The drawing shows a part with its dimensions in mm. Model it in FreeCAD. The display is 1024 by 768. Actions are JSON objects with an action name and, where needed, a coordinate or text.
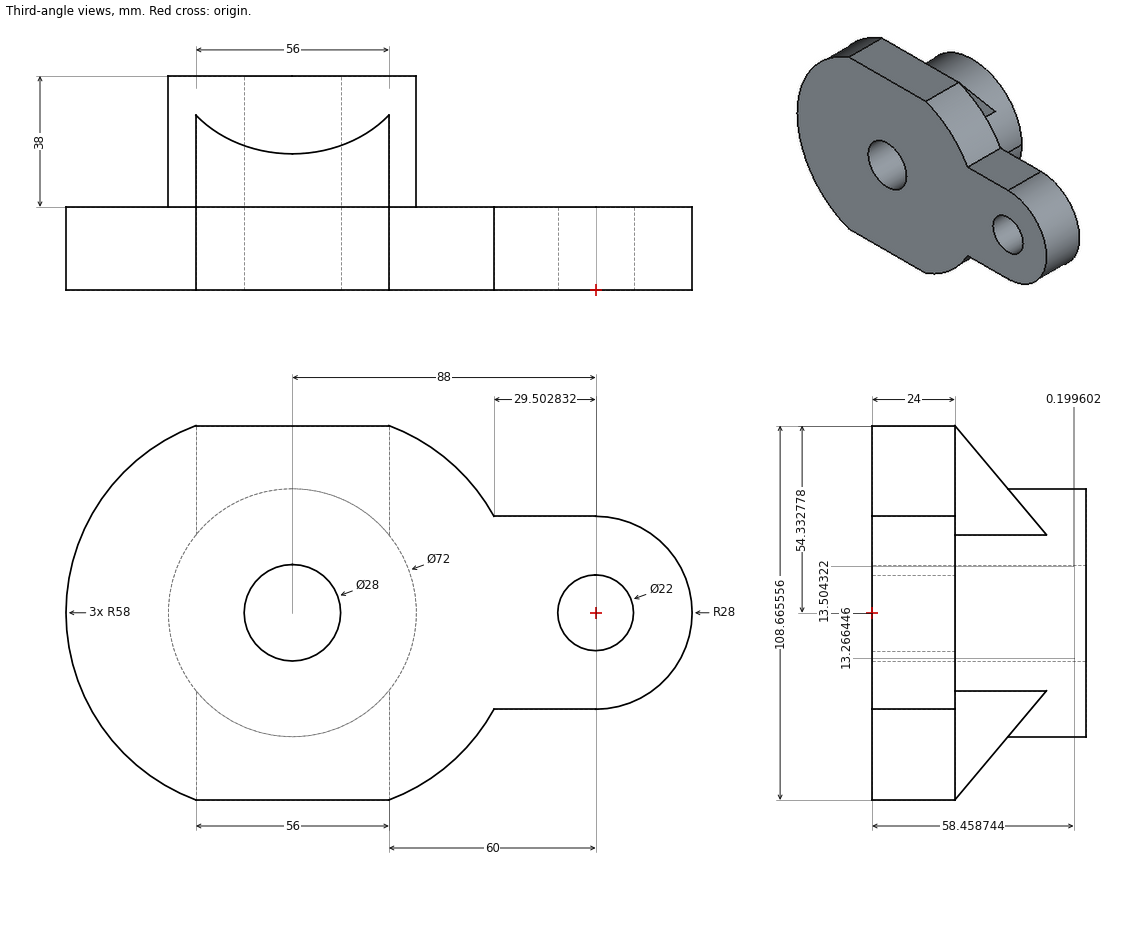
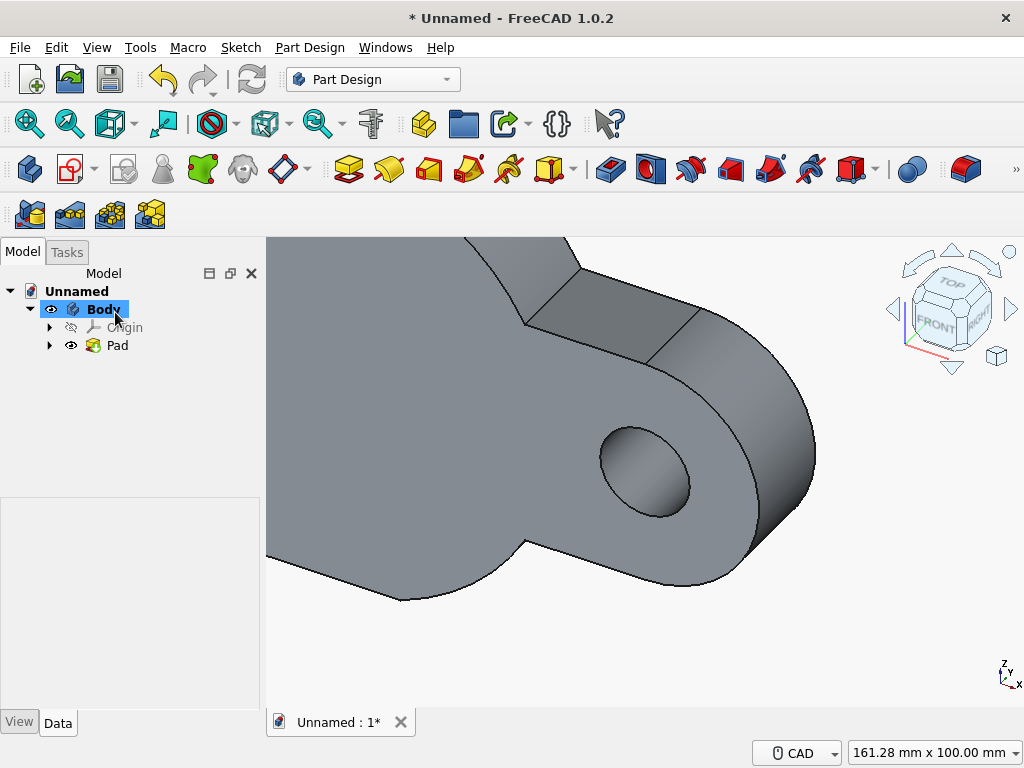
{"action": "left_click", "coordinate": [30, 124]}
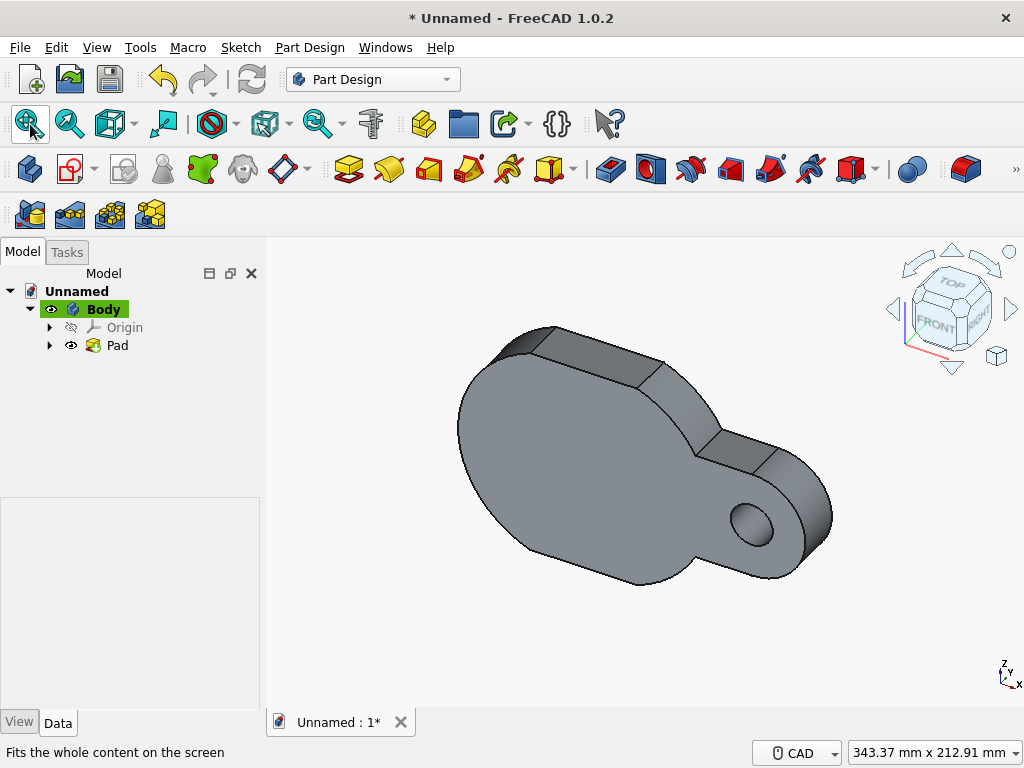
{"action": "key", "text": "4"}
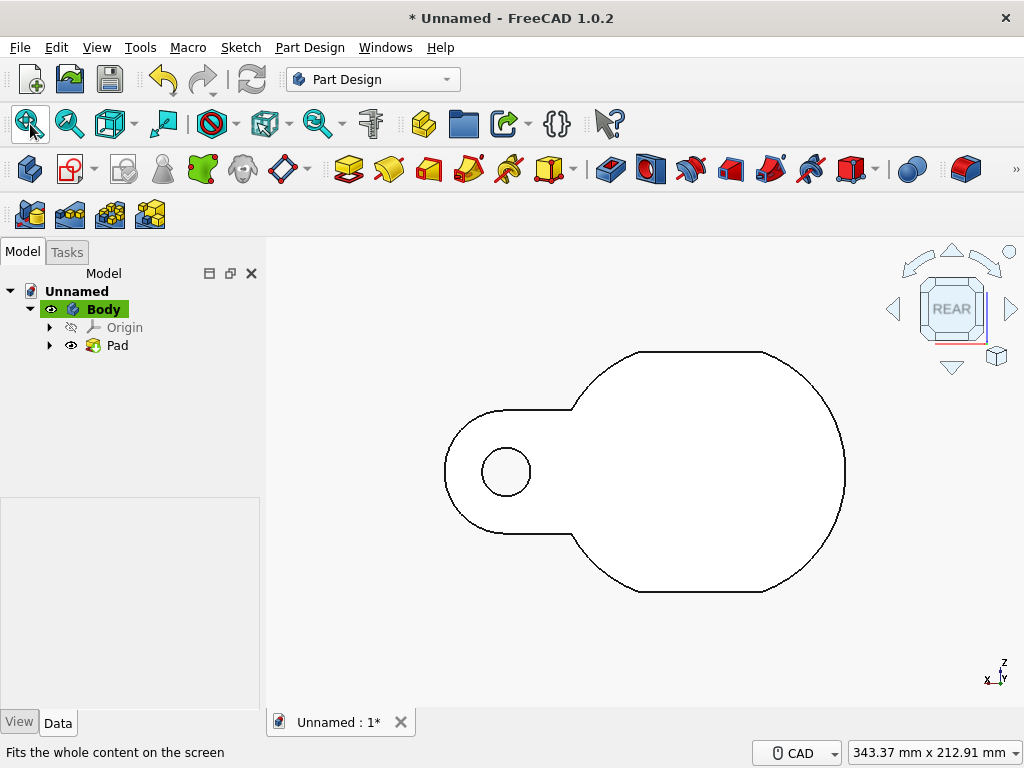
{"action": "left_click", "coordinate": [702, 471]}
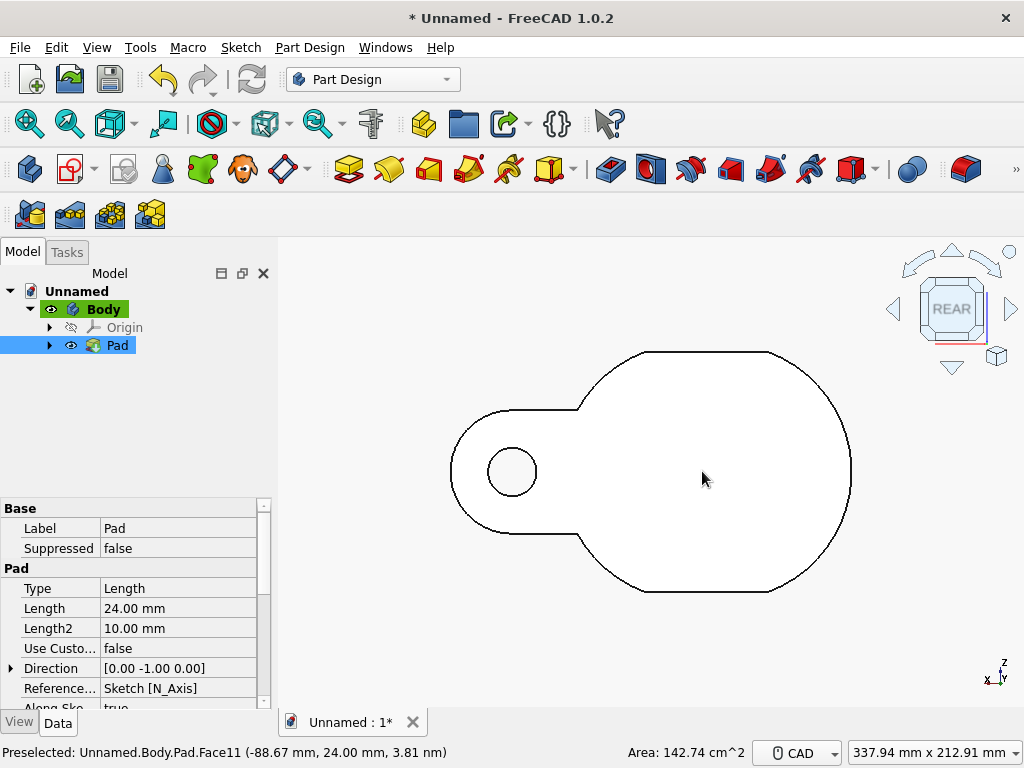
{"action": "left_click", "coordinate": [70, 170]}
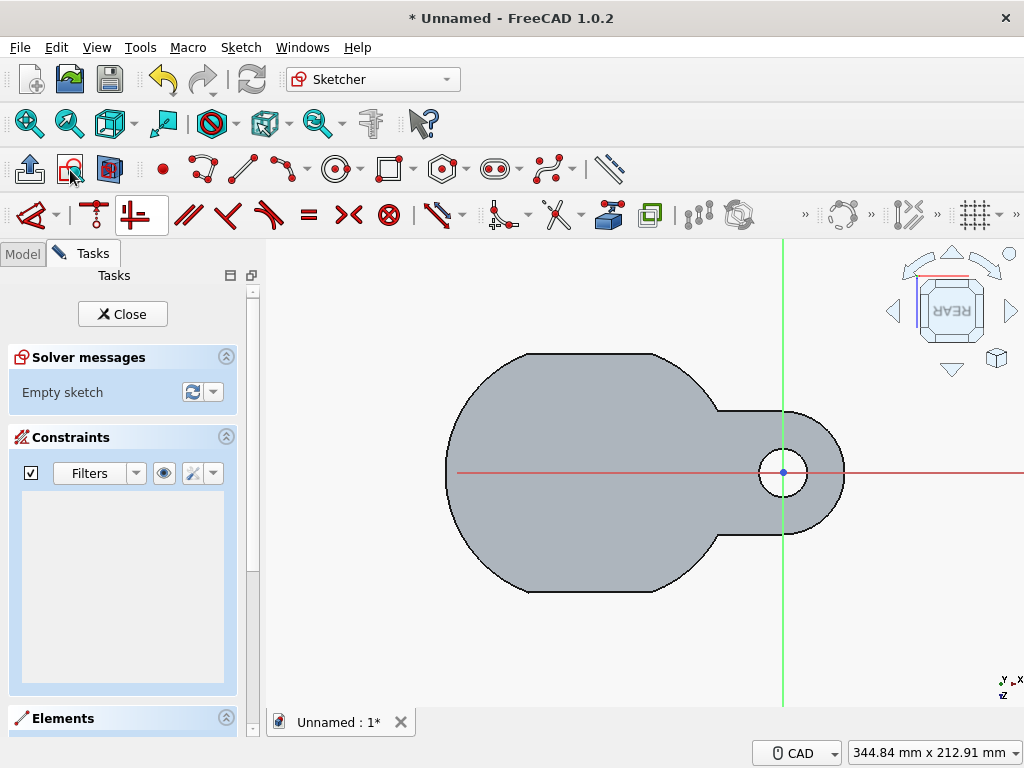
{"action": "scroll", "coordinate": [790, 473], "scroll_direction": "up", "scroll_amount": 2}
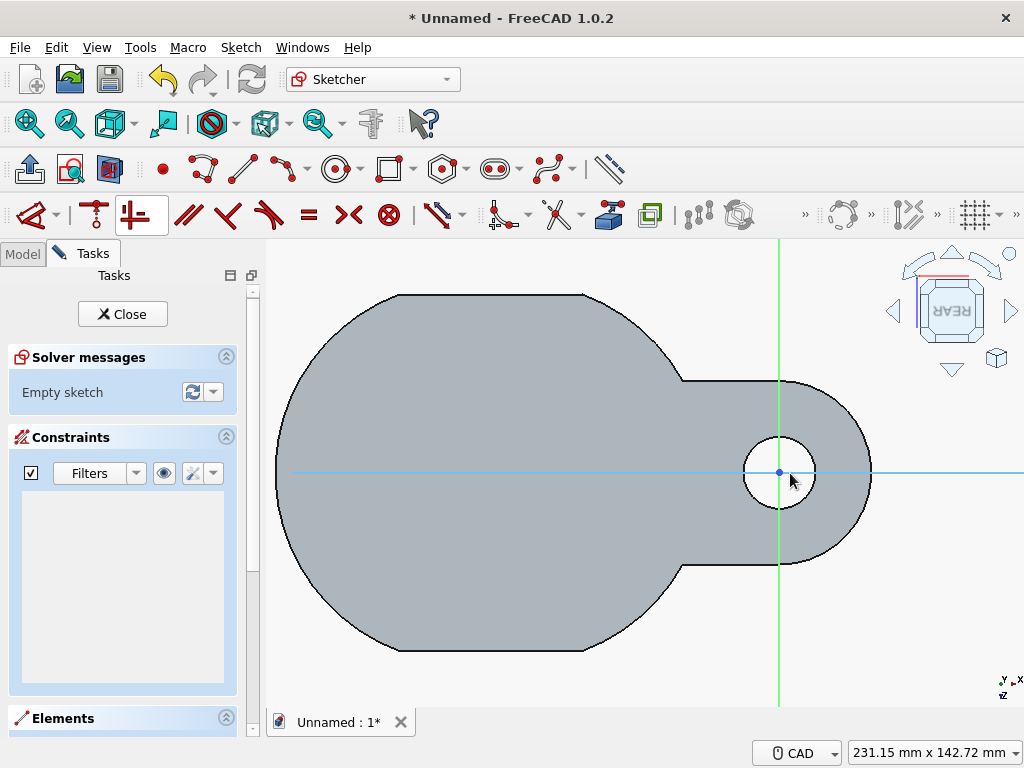
{"action": "left_click", "coordinate": [336, 170]}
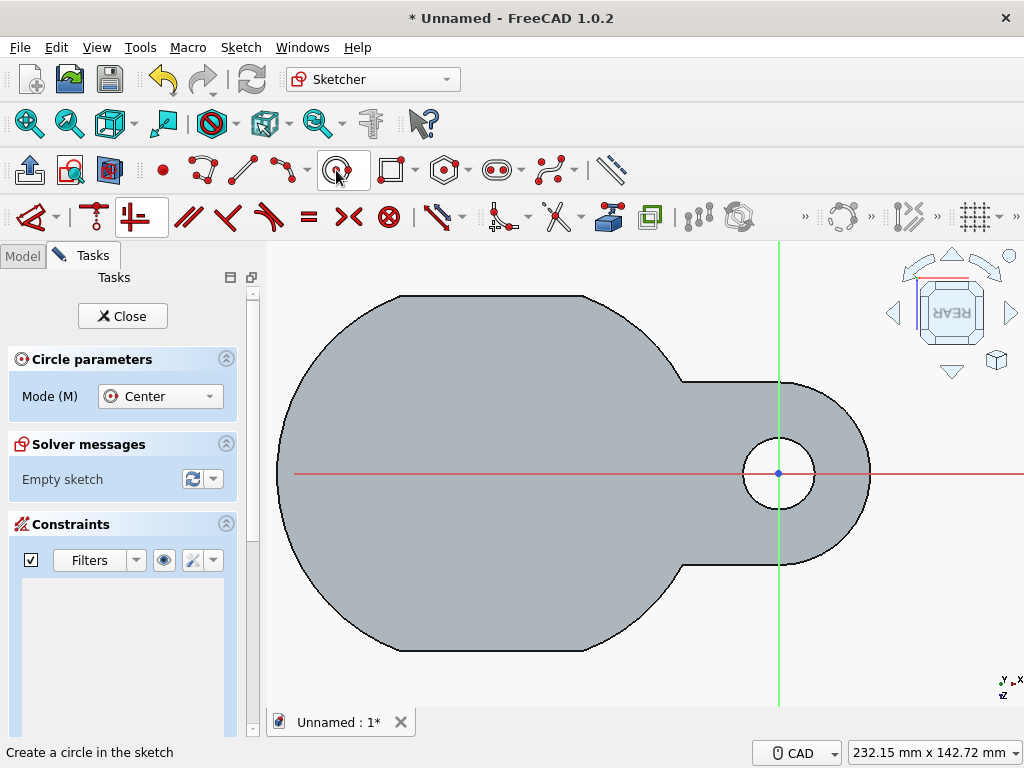
{"action": "left_click", "coordinate": [492, 474]}
{"action": "mouse_move", "coordinate": [575, 391]}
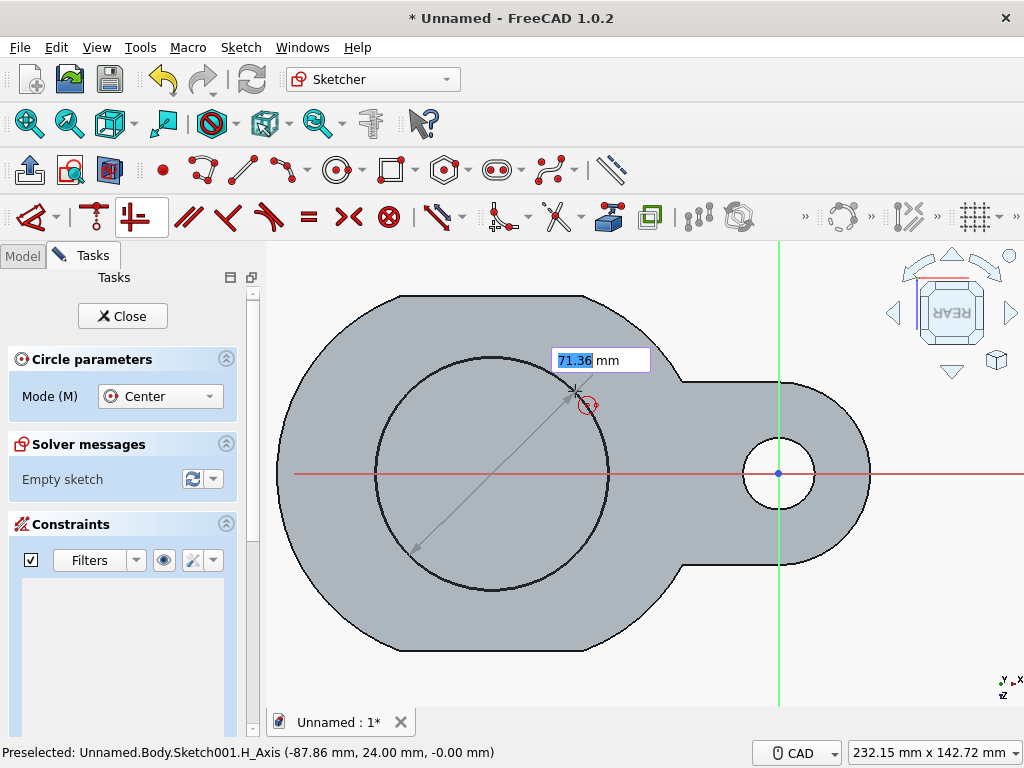
{"action": "type", "text": "72"}
{"action": "key", "text": "Return"}
{"action": "key", "text": "Escape"}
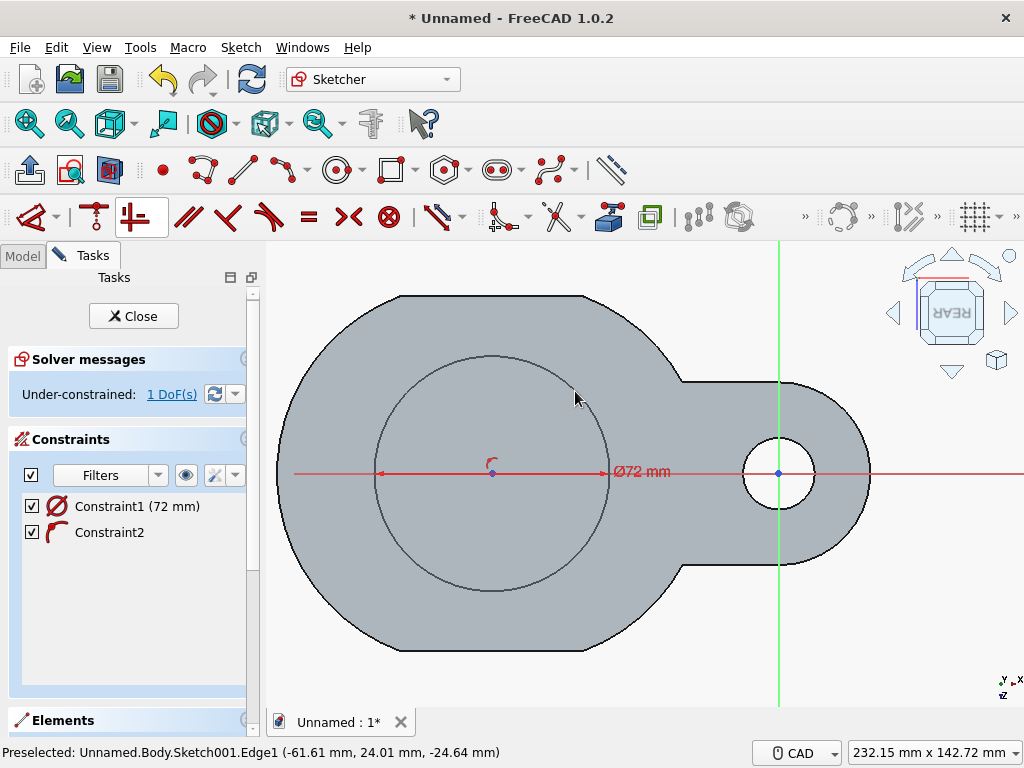
{"action": "left_click", "coordinate": [32, 218]}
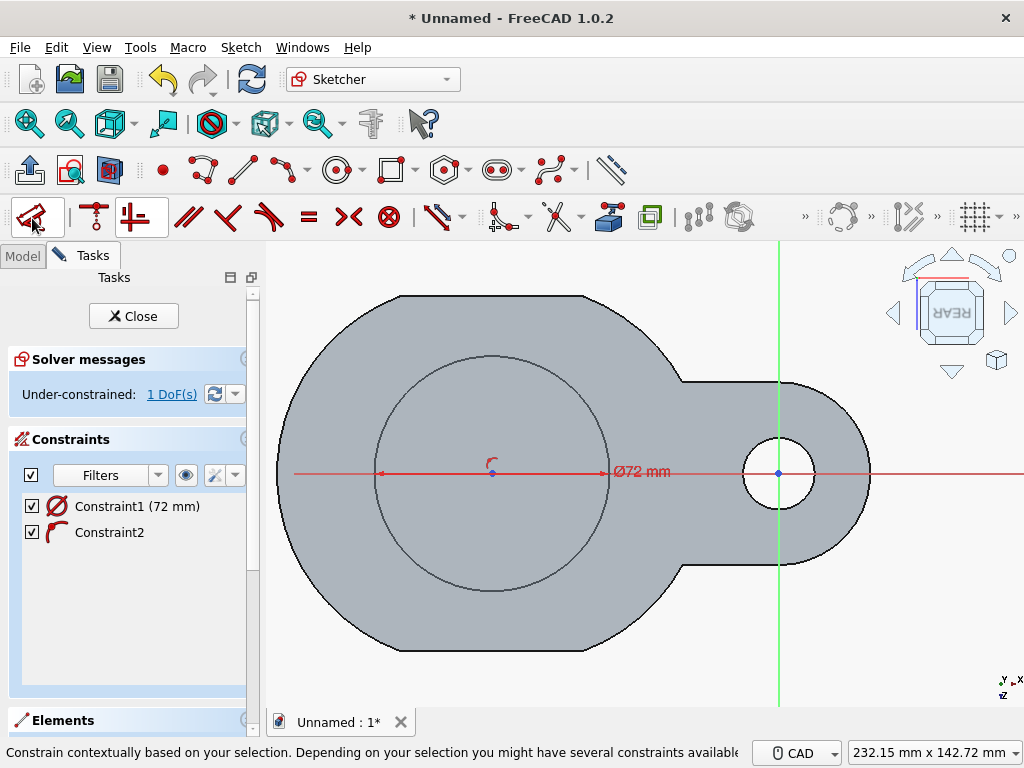
{"action": "left_click", "coordinate": [492, 474]}
{"action": "left_click", "coordinate": [635, 508]}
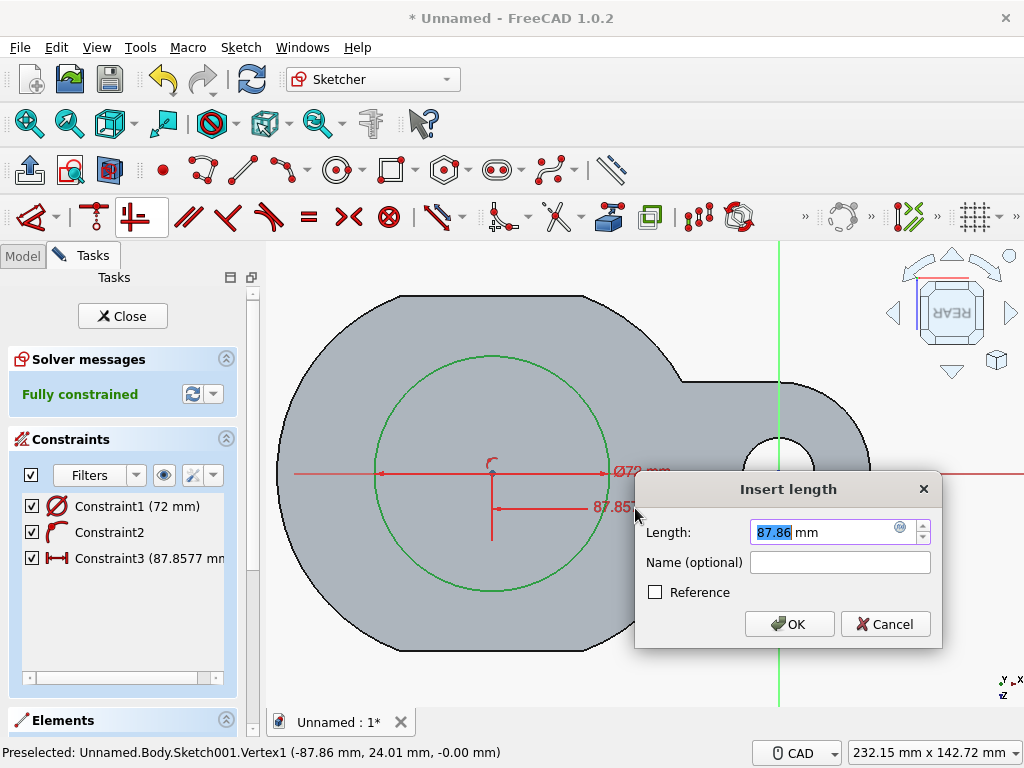
{"action": "type", "text": "88"}
{"action": "key", "text": "Return"}
{"action": "key", "text": "Escape"}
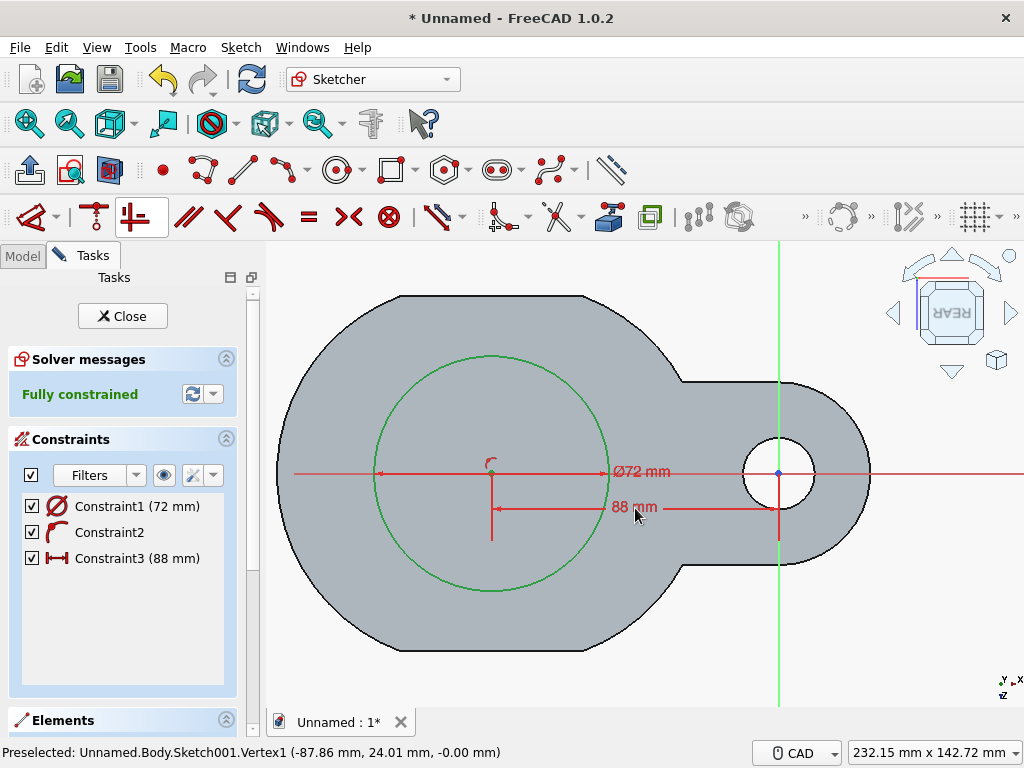
{"action": "left_click", "coordinate": [123, 316]}